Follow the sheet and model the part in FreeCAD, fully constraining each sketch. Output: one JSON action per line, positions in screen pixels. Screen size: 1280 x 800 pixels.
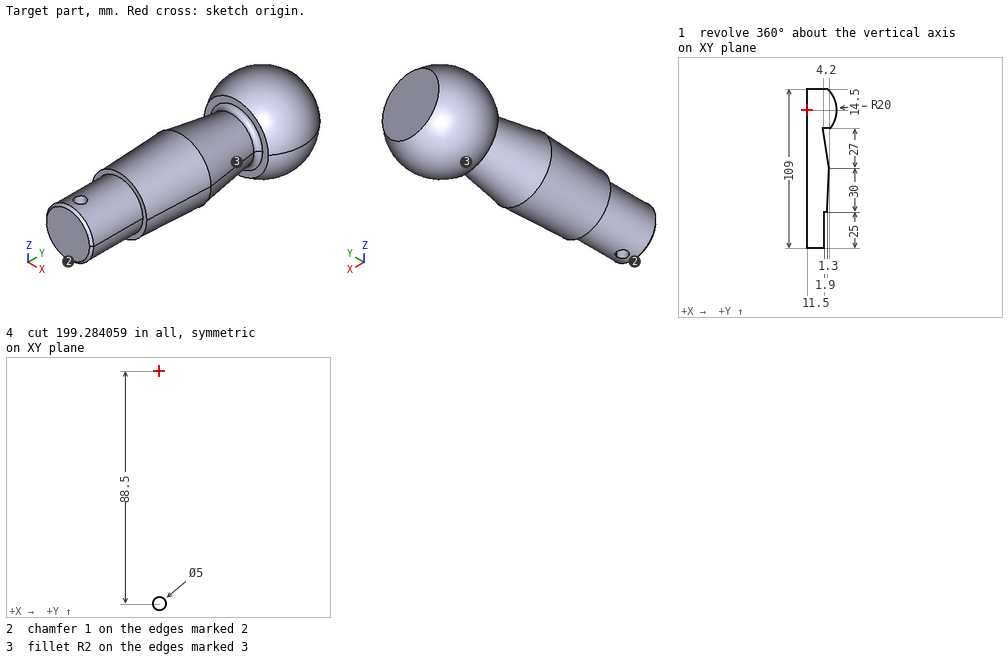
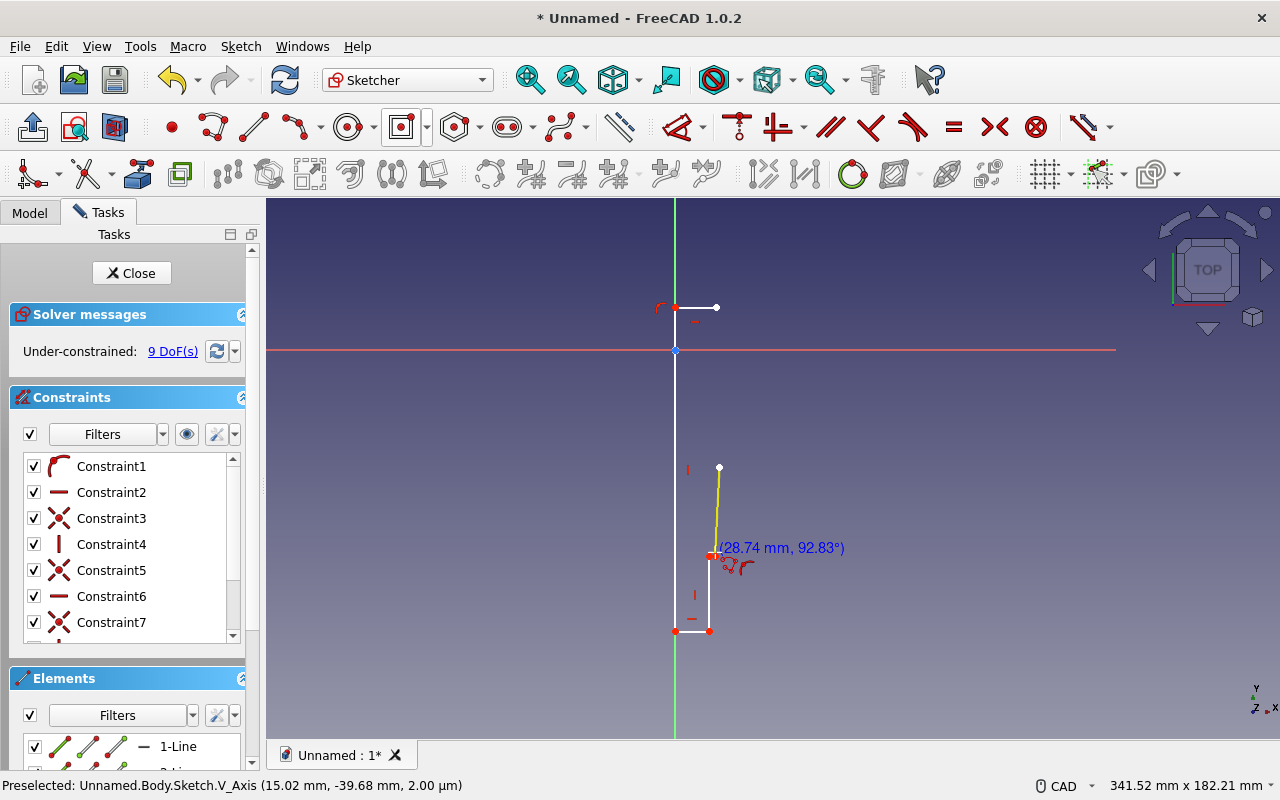
{"action": "left_click", "coordinate": [706, 387]}
{"action": "left_click", "coordinate": [722, 387]}
{"action": "right_click", "coordinate": [722, 387]}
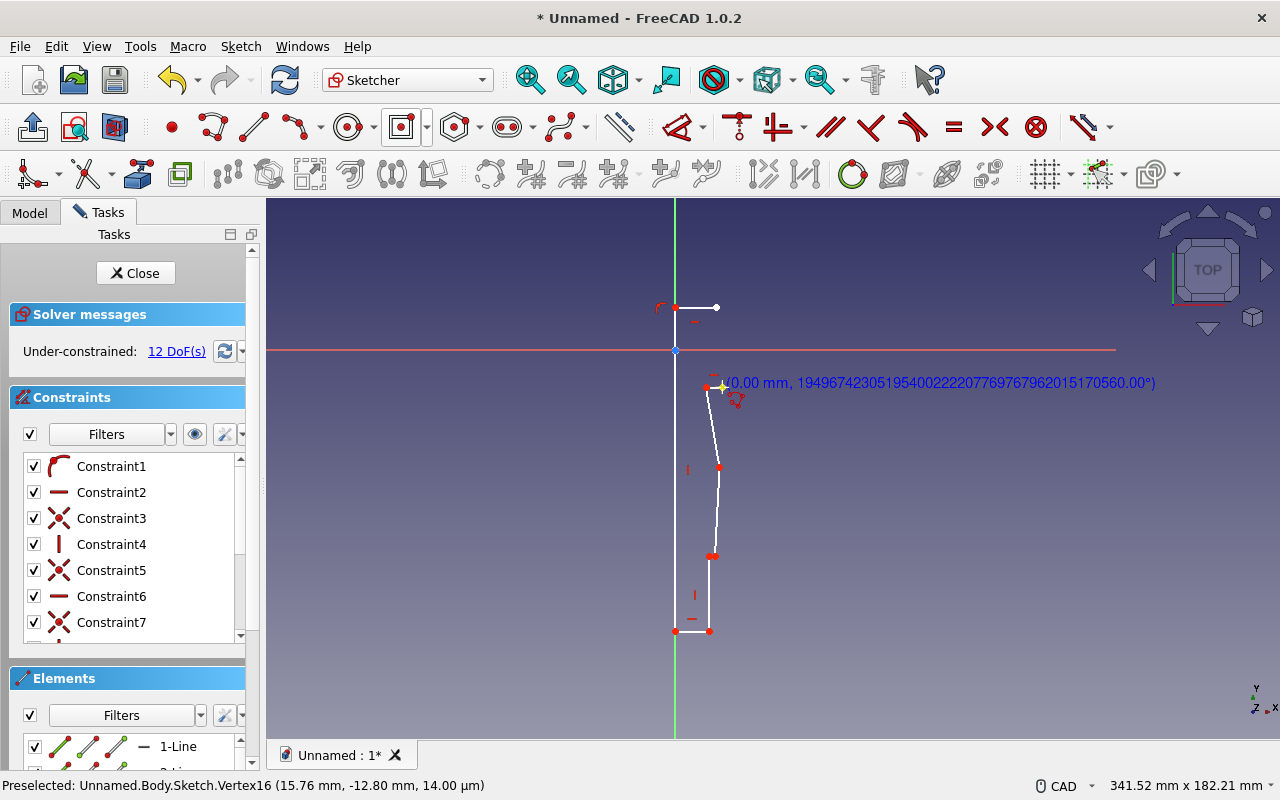
{"action": "left_click", "coordinate": [294, 128]}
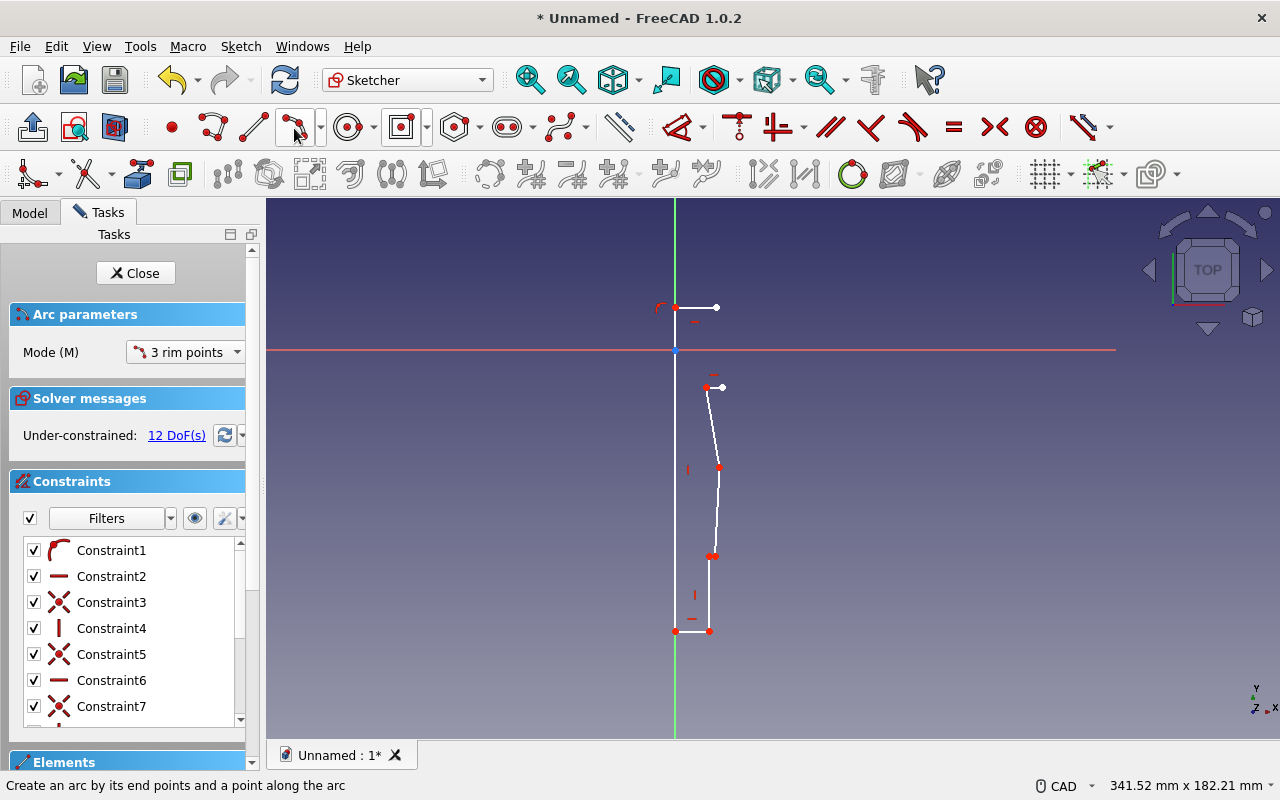
{"action": "scroll", "coordinate": [722, 387], "scroll_direction": "up", "scroll_amount": 4}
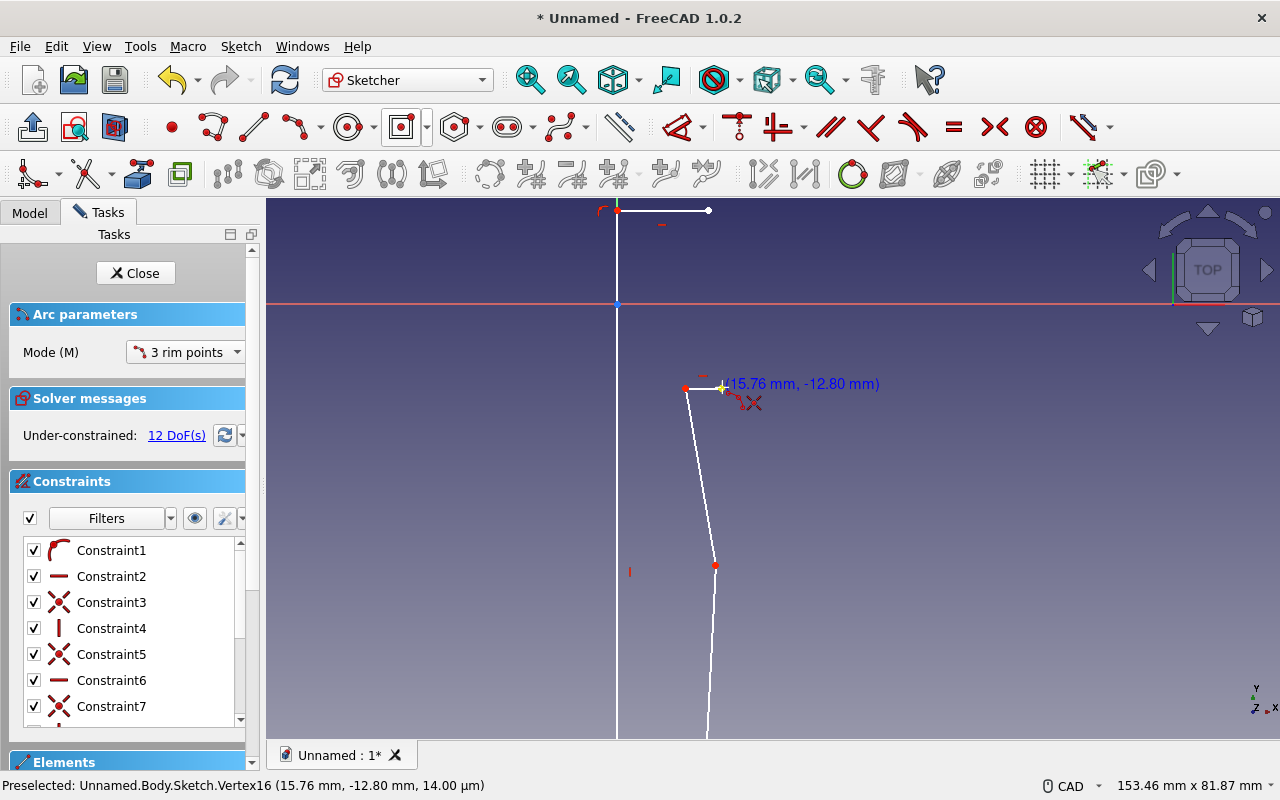
{"action": "left_click", "coordinate": [721, 389]}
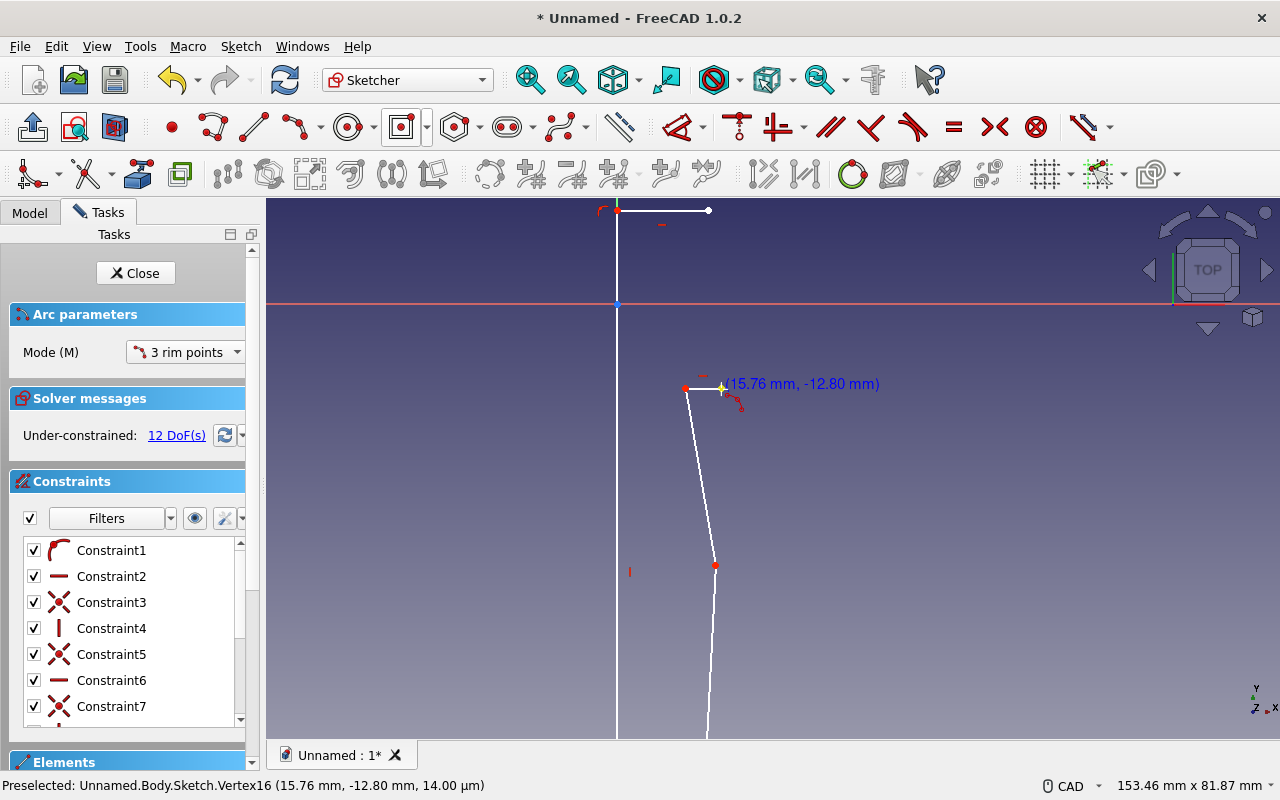
{"action": "scroll", "coordinate": [722, 387], "scroll_direction": "down", "scroll_amount": 4}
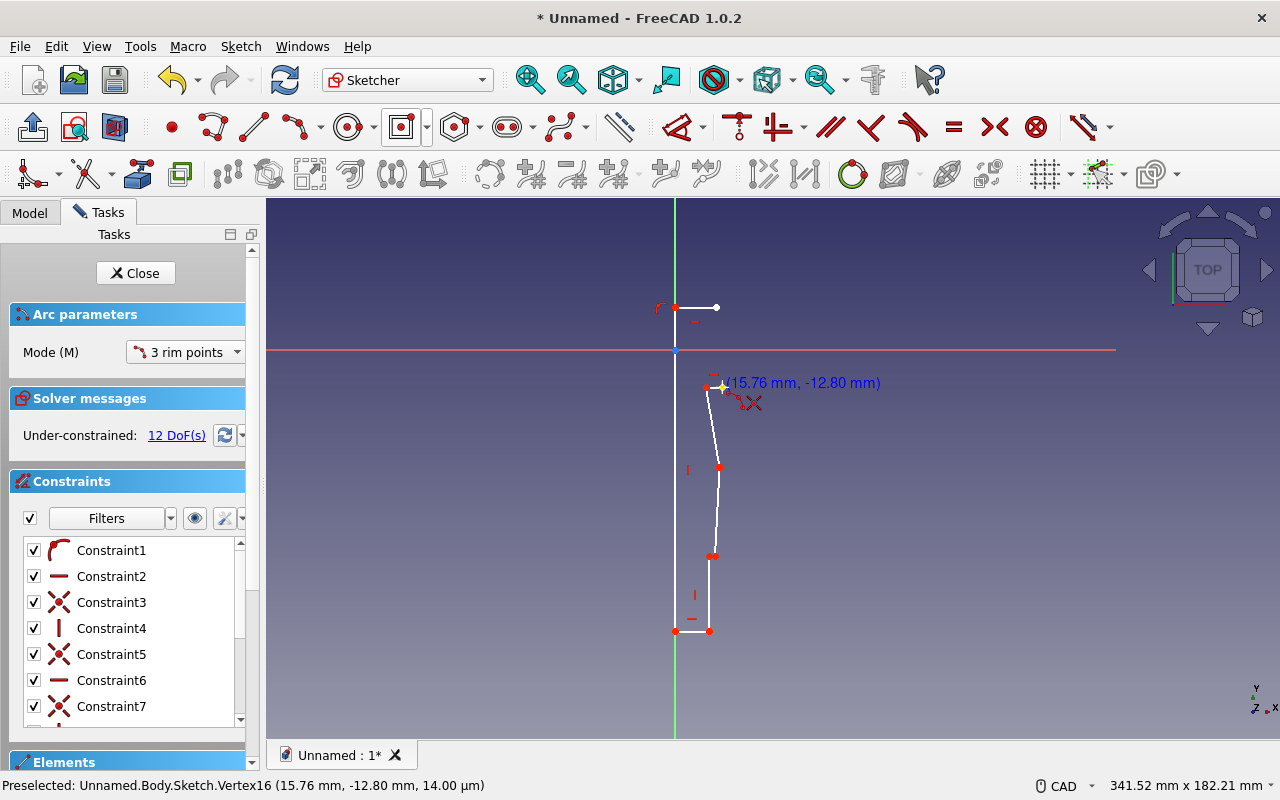
{"action": "left_click", "coordinate": [716, 308]}
{"action": "left_click", "coordinate": [733, 364]}
{"action": "key", "text": "Escape"}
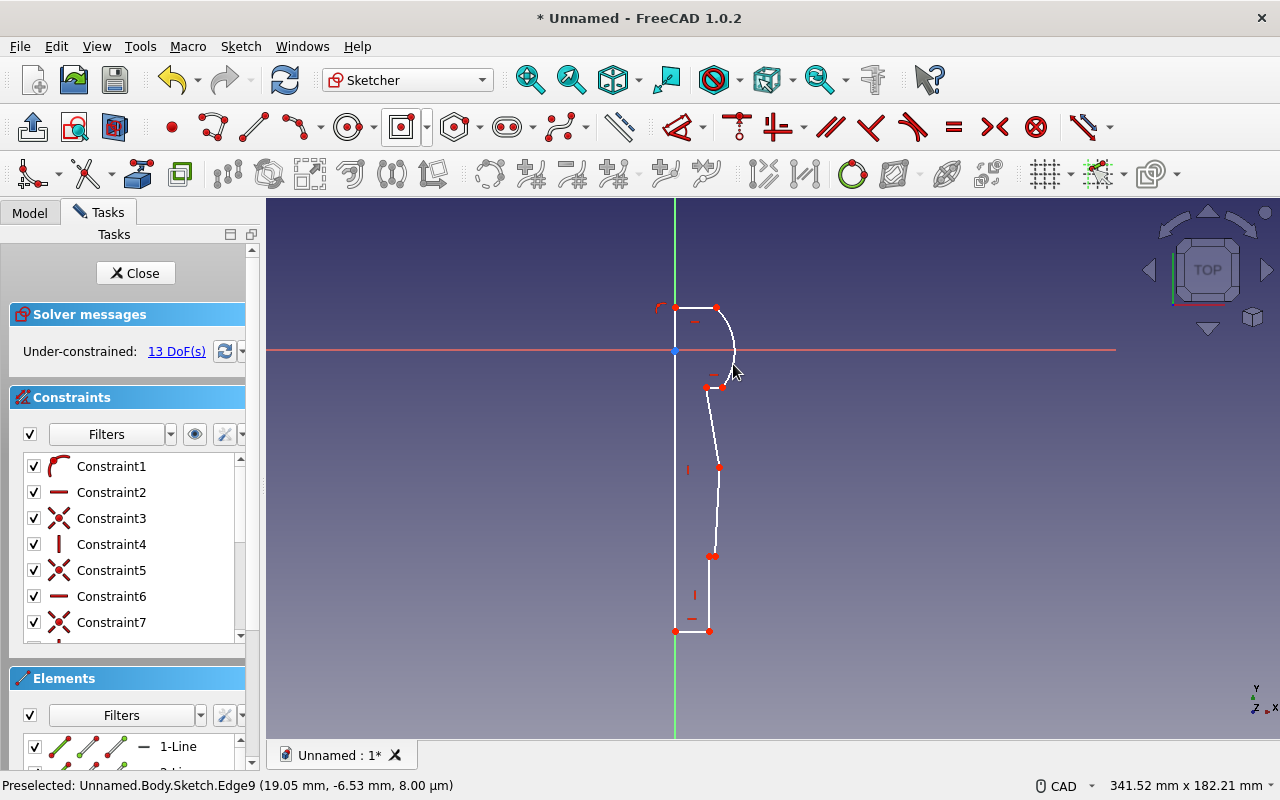
{"action": "scroll", "coordinate": [712, 556], "scroll_direction": "up", "scroll_amount": 8}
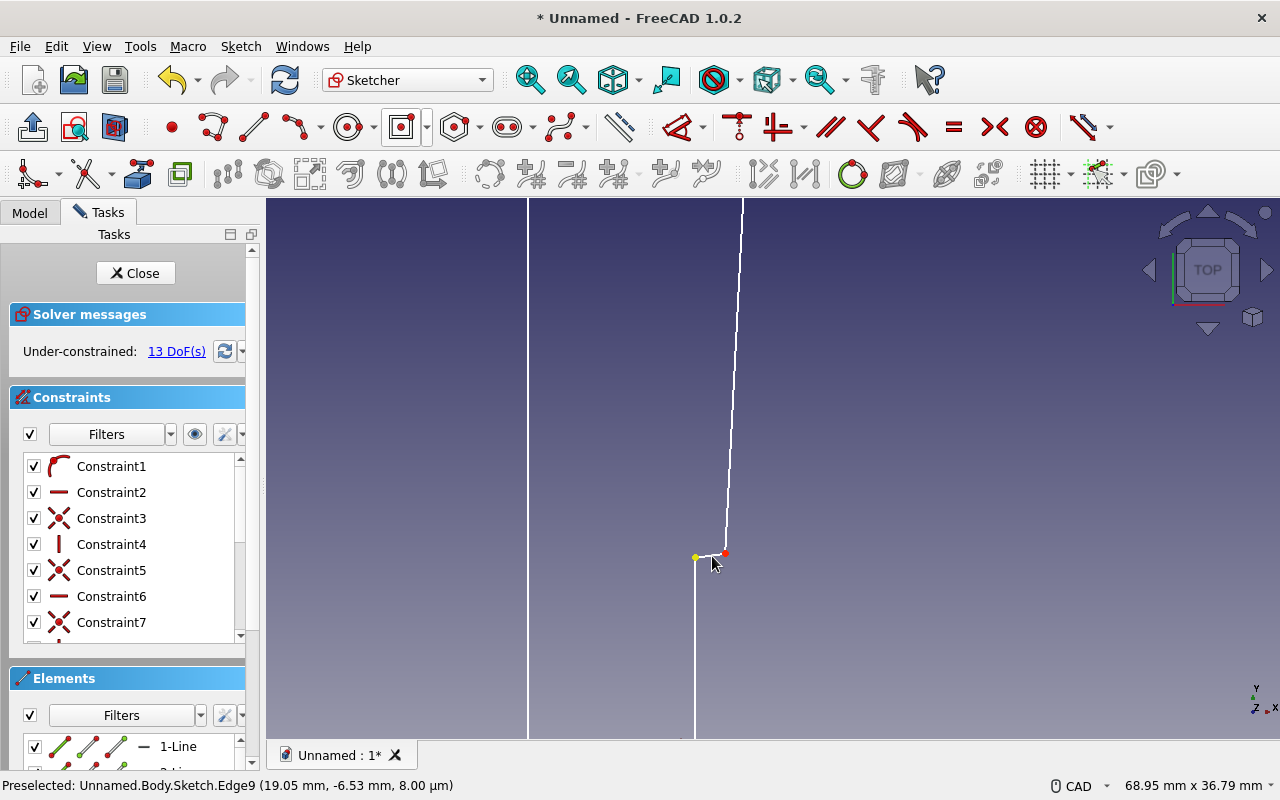
{"action": "left_click", "coordinate": [710, 556]}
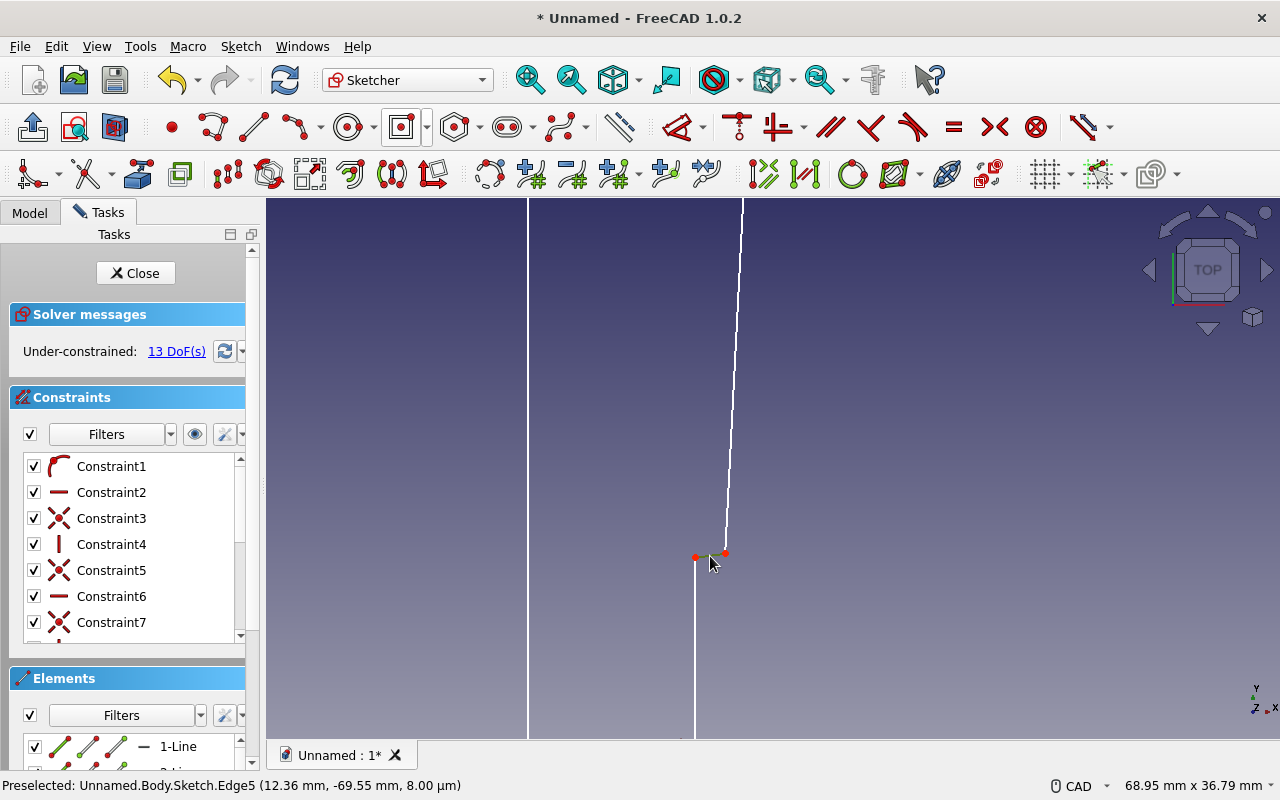
{"action": "left_click", "coordinate": [804, 128]}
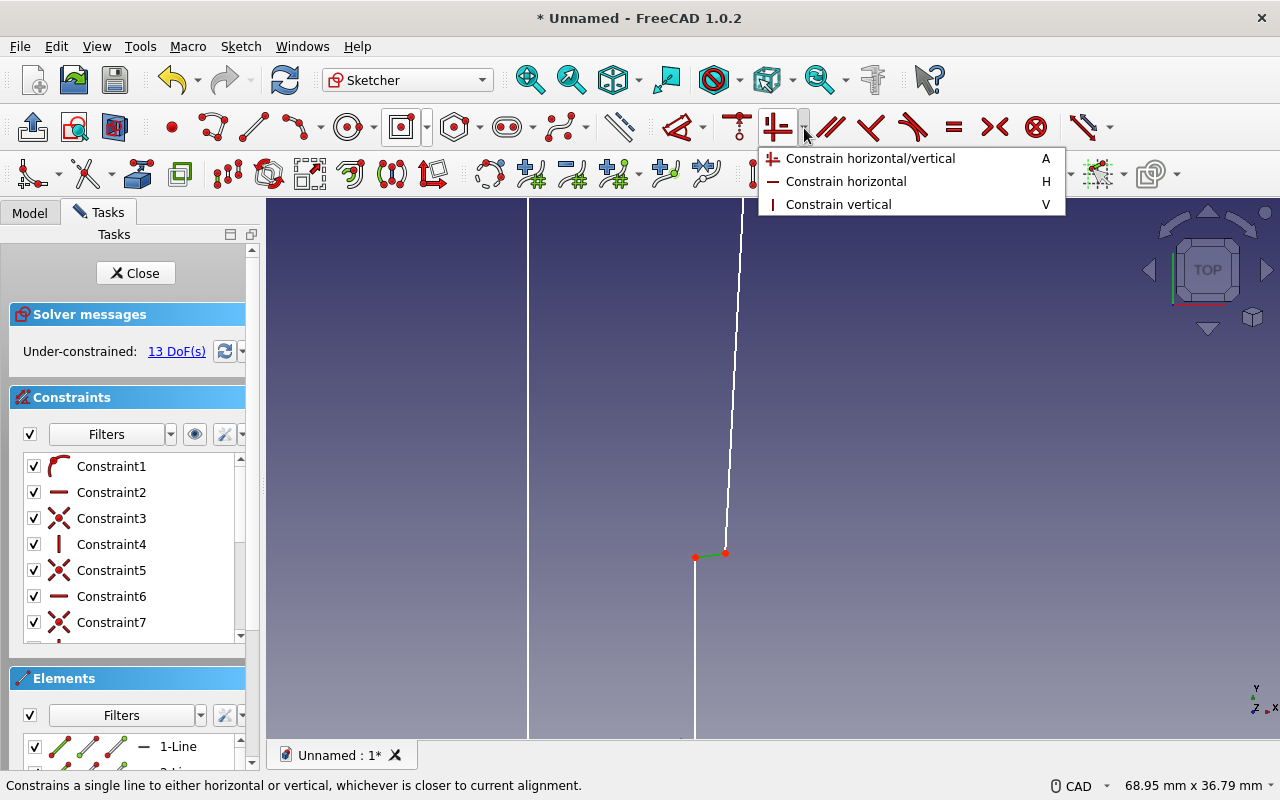
{"action": "left_click", "coordinate": [912, 182]}